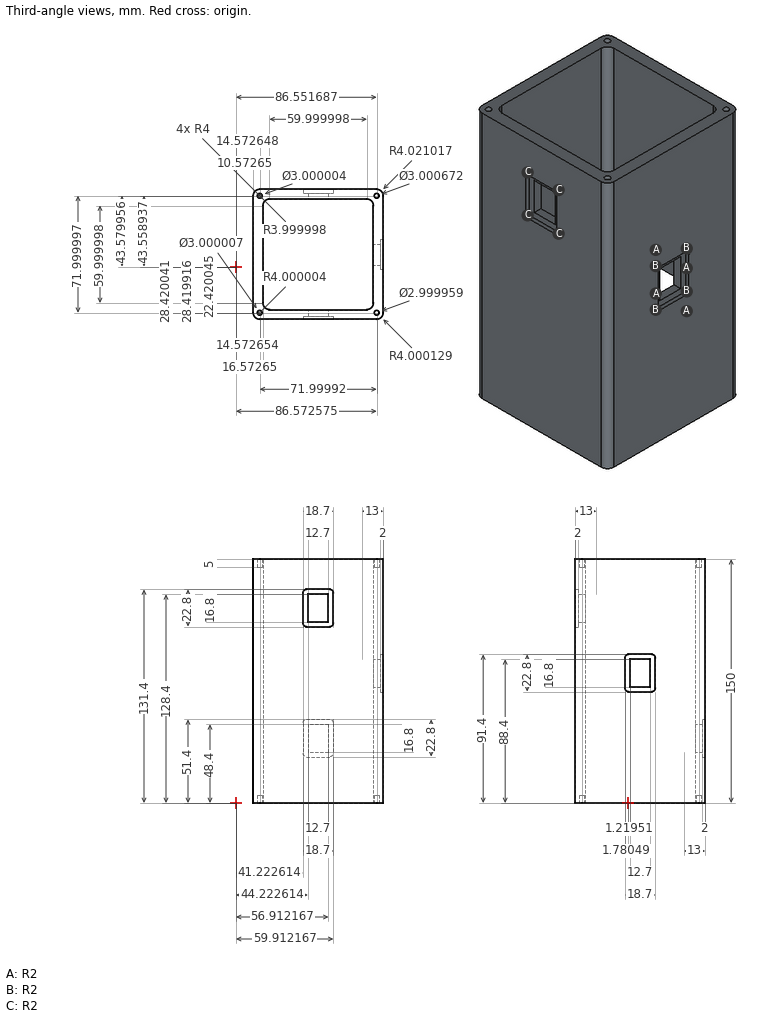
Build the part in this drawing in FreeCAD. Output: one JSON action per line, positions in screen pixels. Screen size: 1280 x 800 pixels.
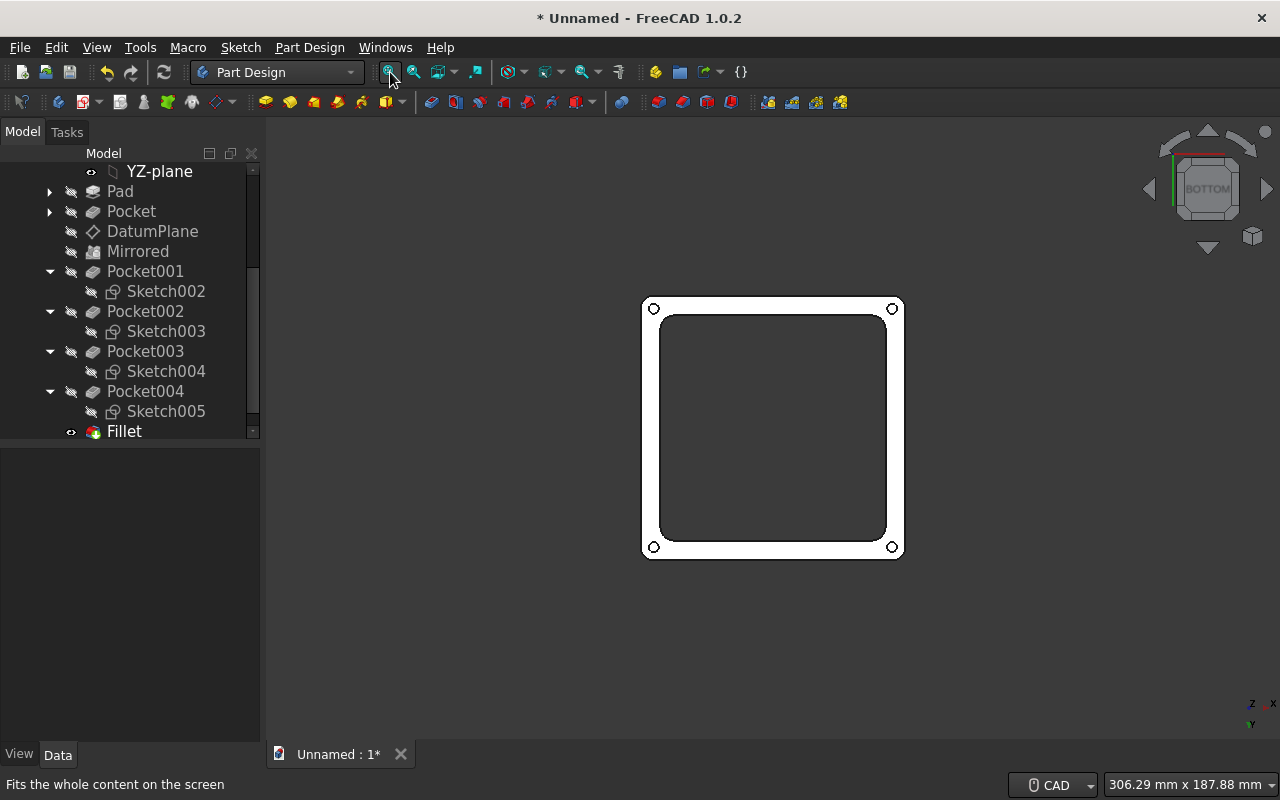
{"action": "key", "text": "0"}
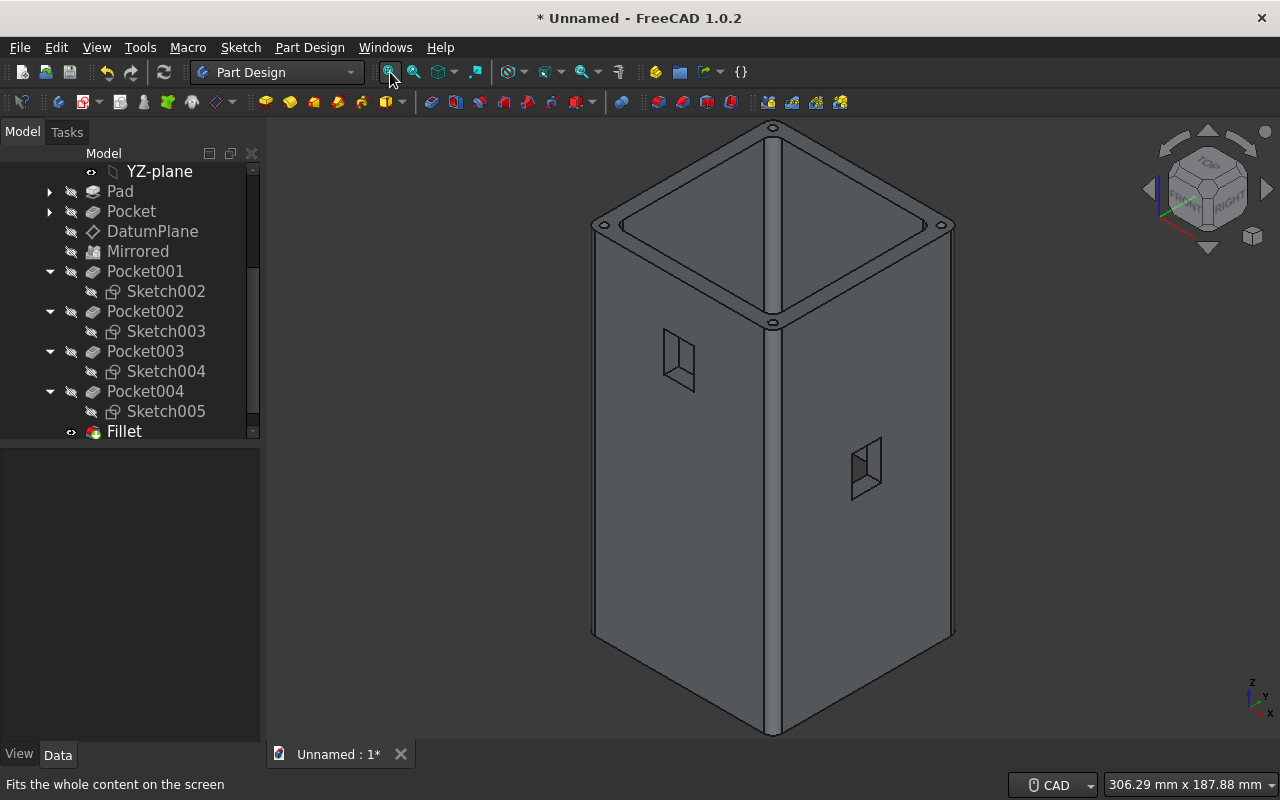
{"action": "left_click", "coordinate": [390, 72]}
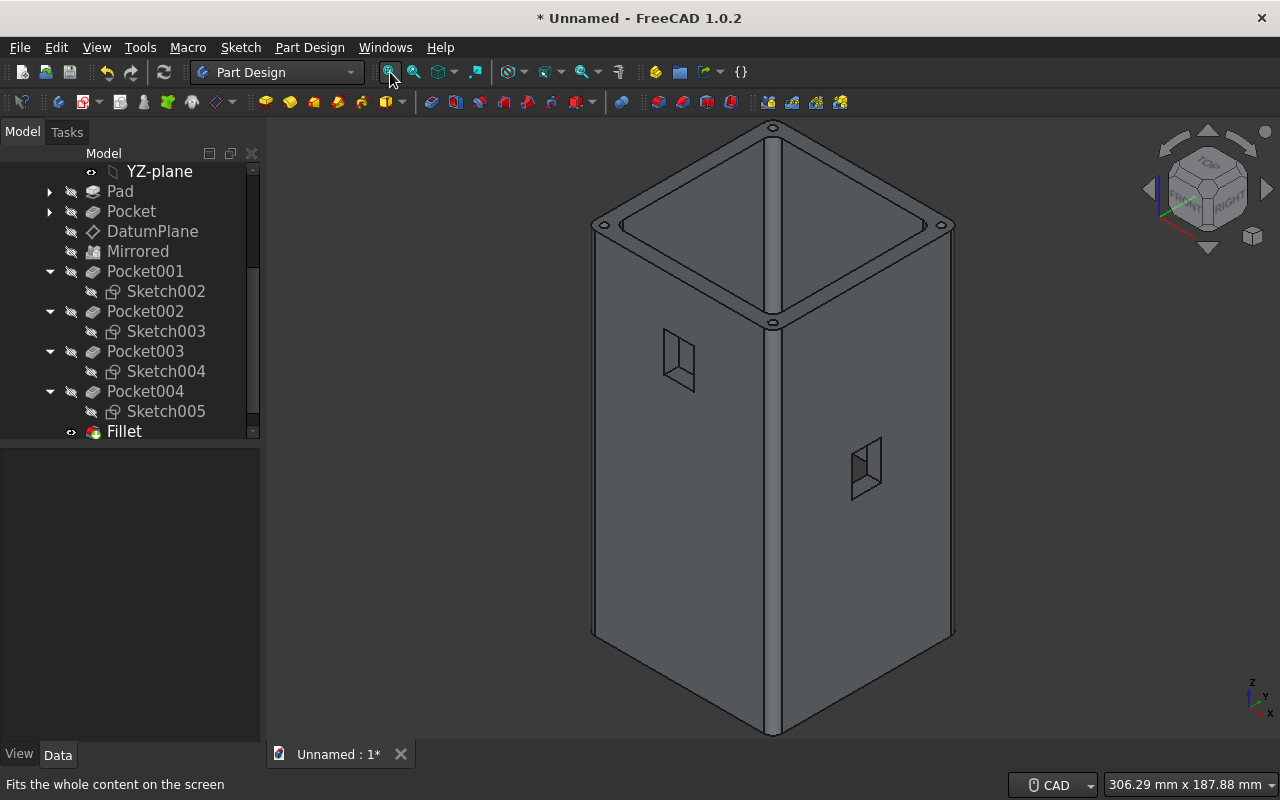
{"action": "left_click", "coordinate": [867, 597]}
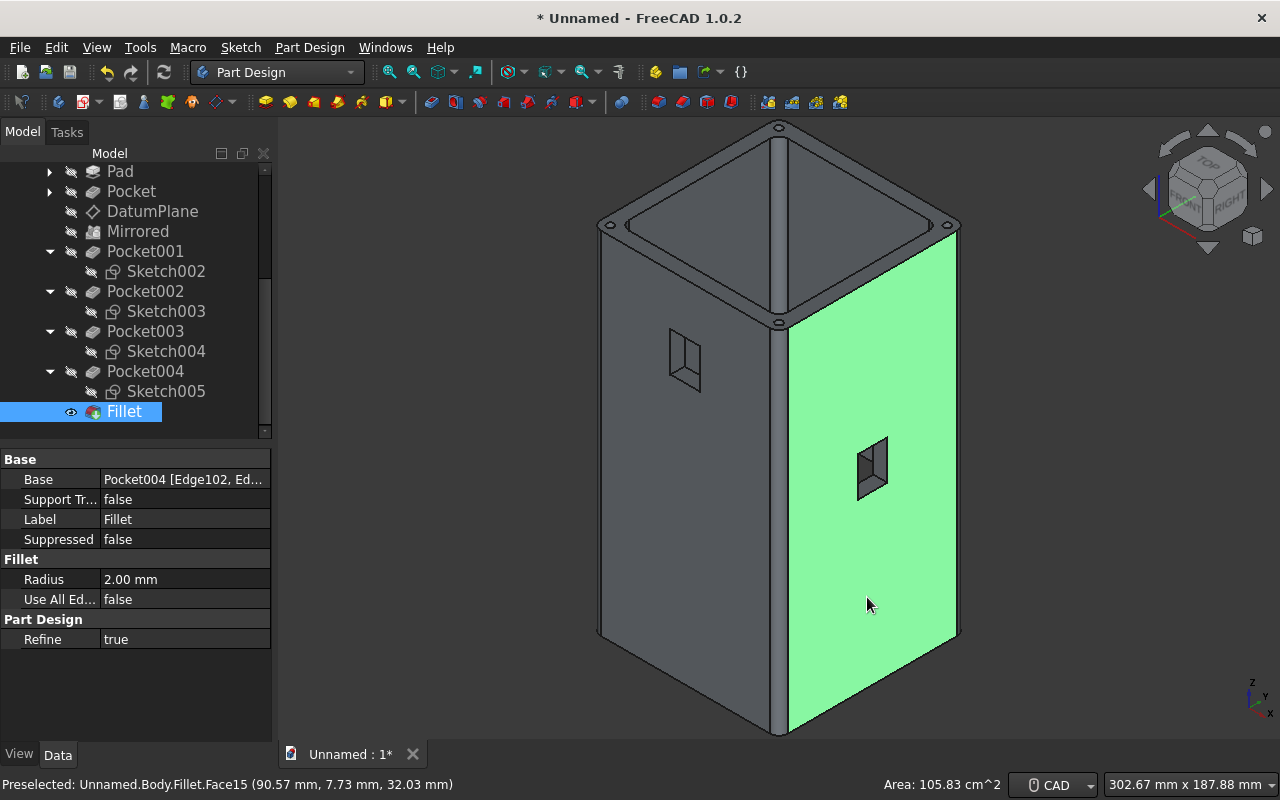
{"action": "left_click", "coordinate": [84, 102]}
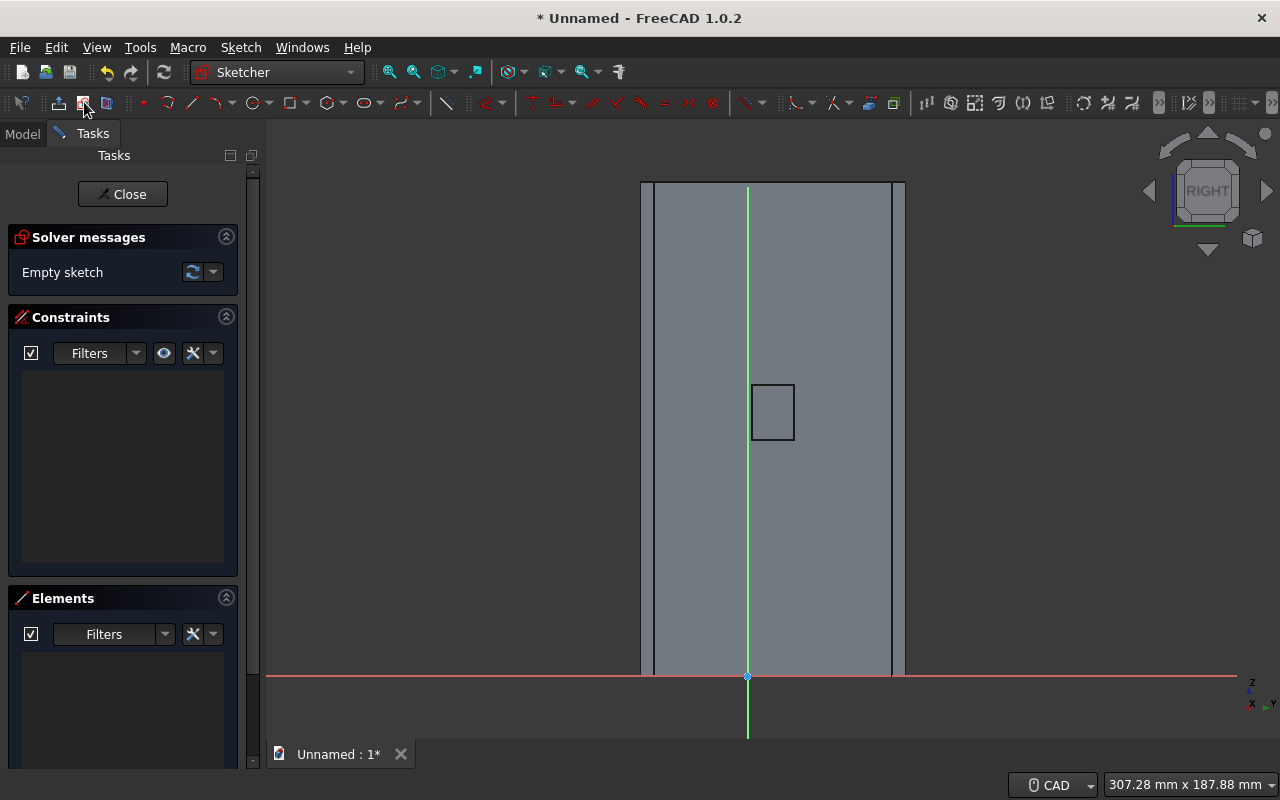
{"action": "scroll", "coordinate": [790, 408], "scroll_direction": "up", "scroll_amount": 8}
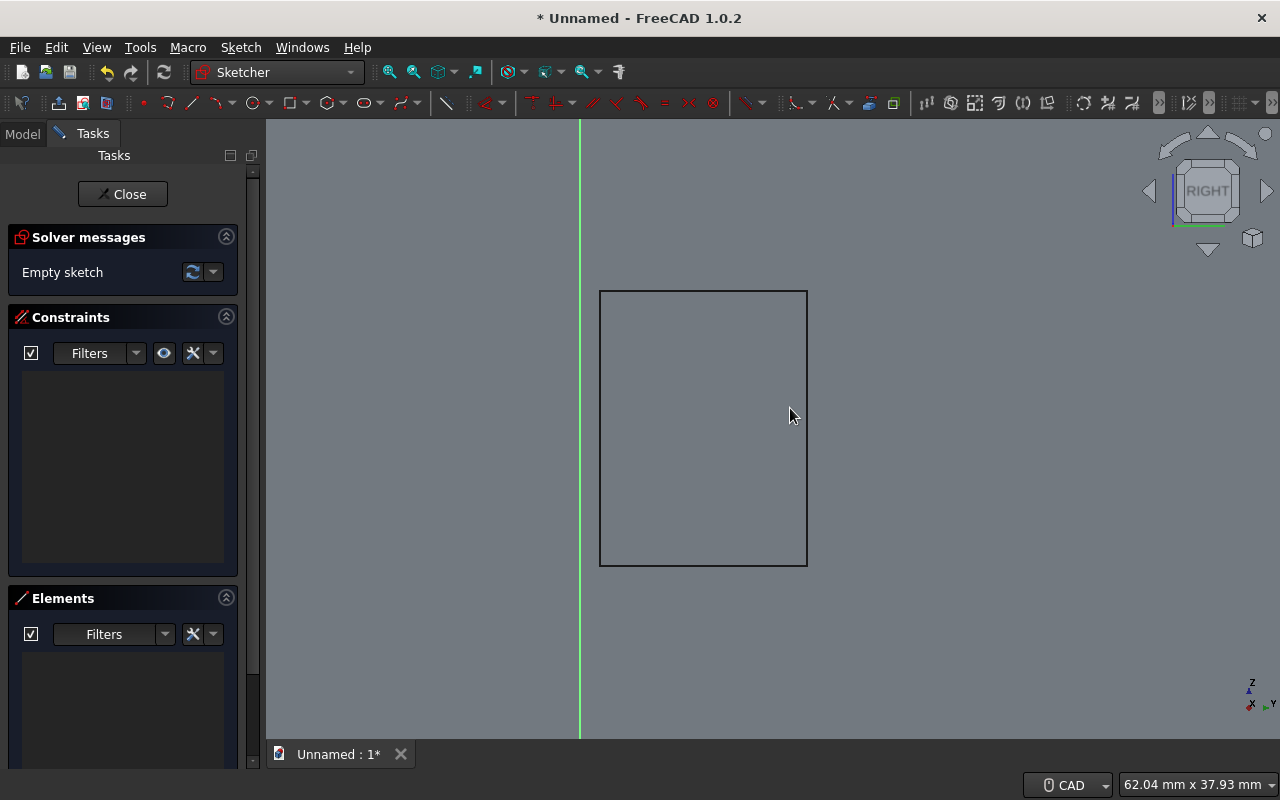
{"action": "left_click", "coordinate": [290, 104]}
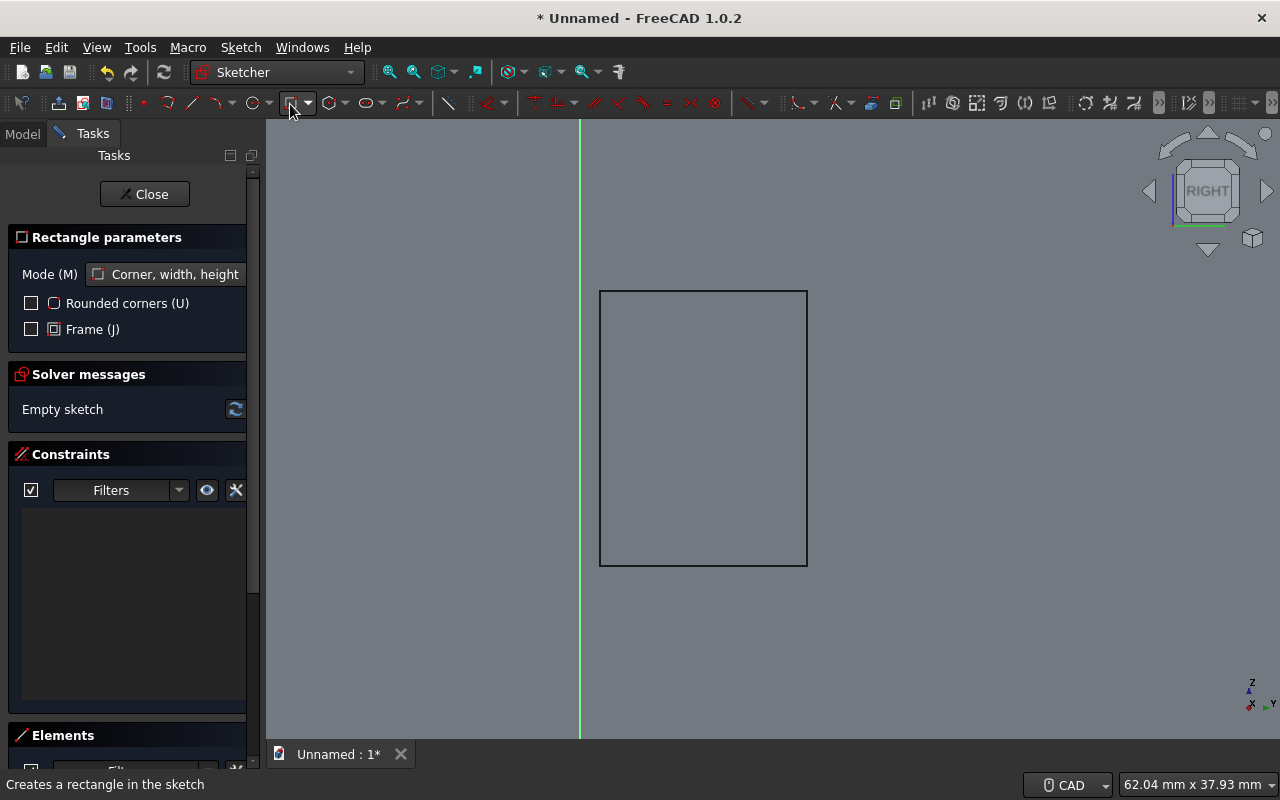
{"action": "left_click", "coordinate": [551, 242]}
{"action": "left_click", "coordinate": [856, 615]}
{"action": "key", "text": "Escape"}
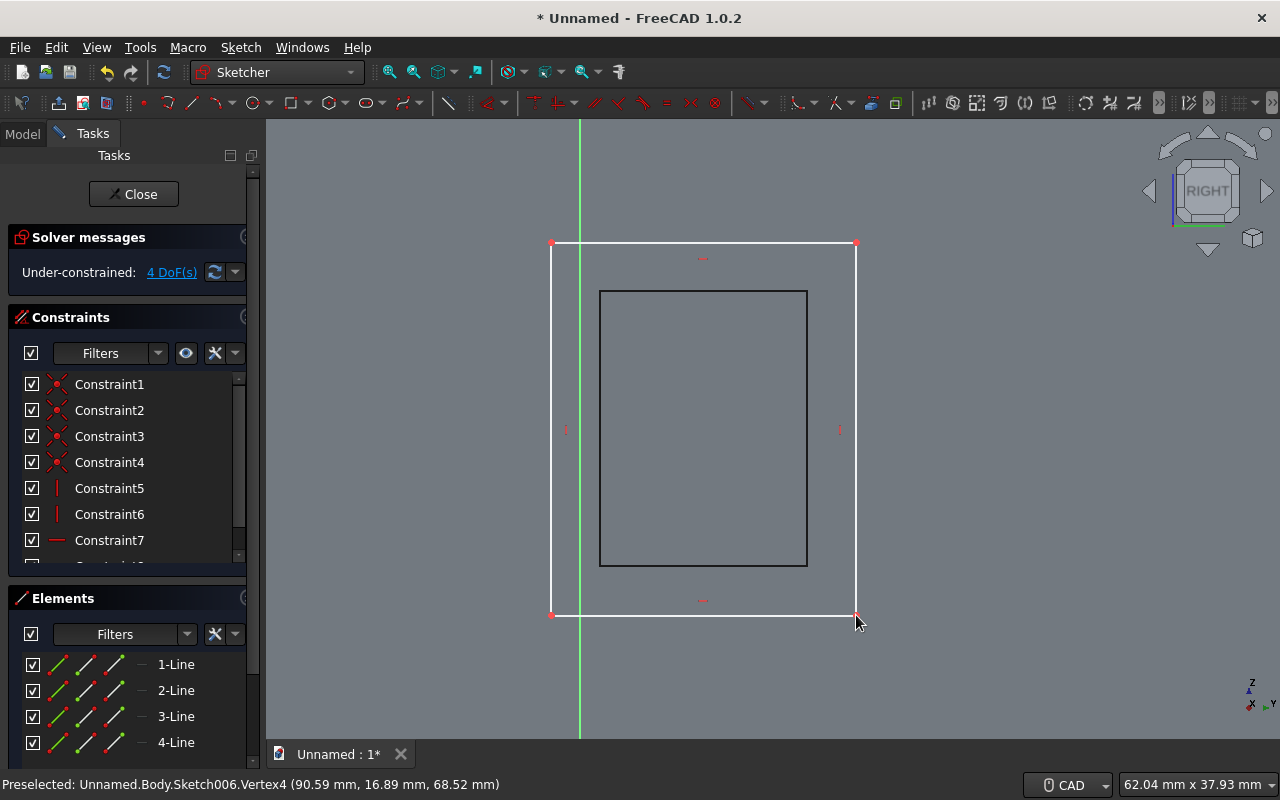
{"action": "left_click", "coordinate": [488, 104]}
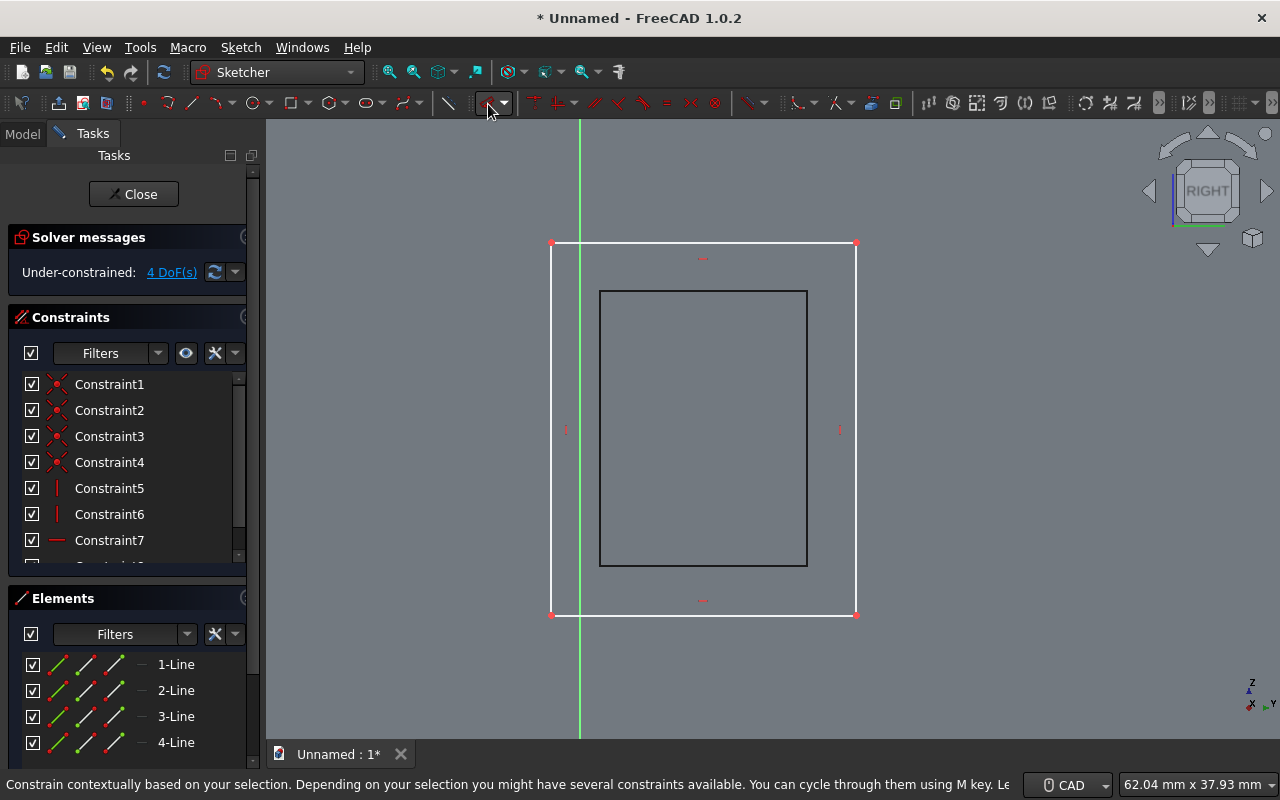
{"action": "left_click", "coordinate": [551, 355]}
{"action": "left_click", "coordinate": [517, 429]}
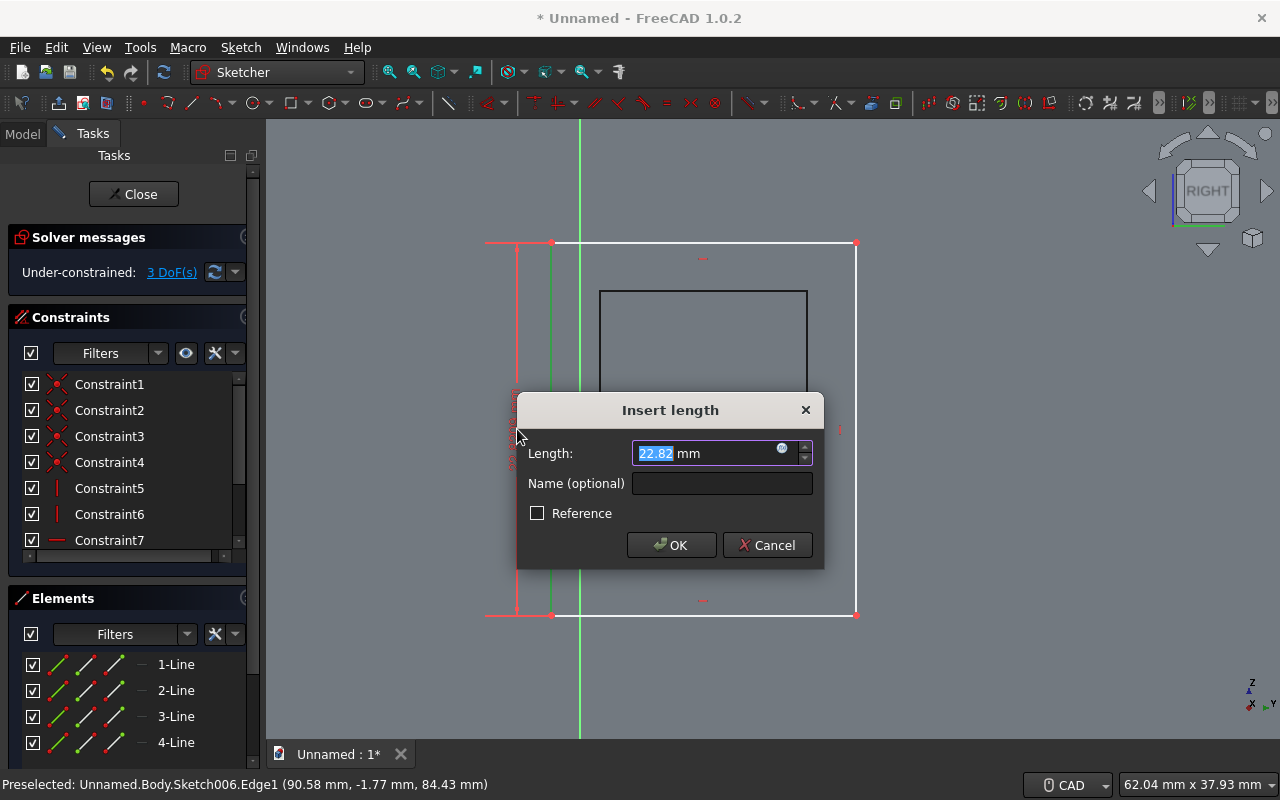
{"action": "type", "text": "22.8"}
{"action": "key", "text": "Return"}